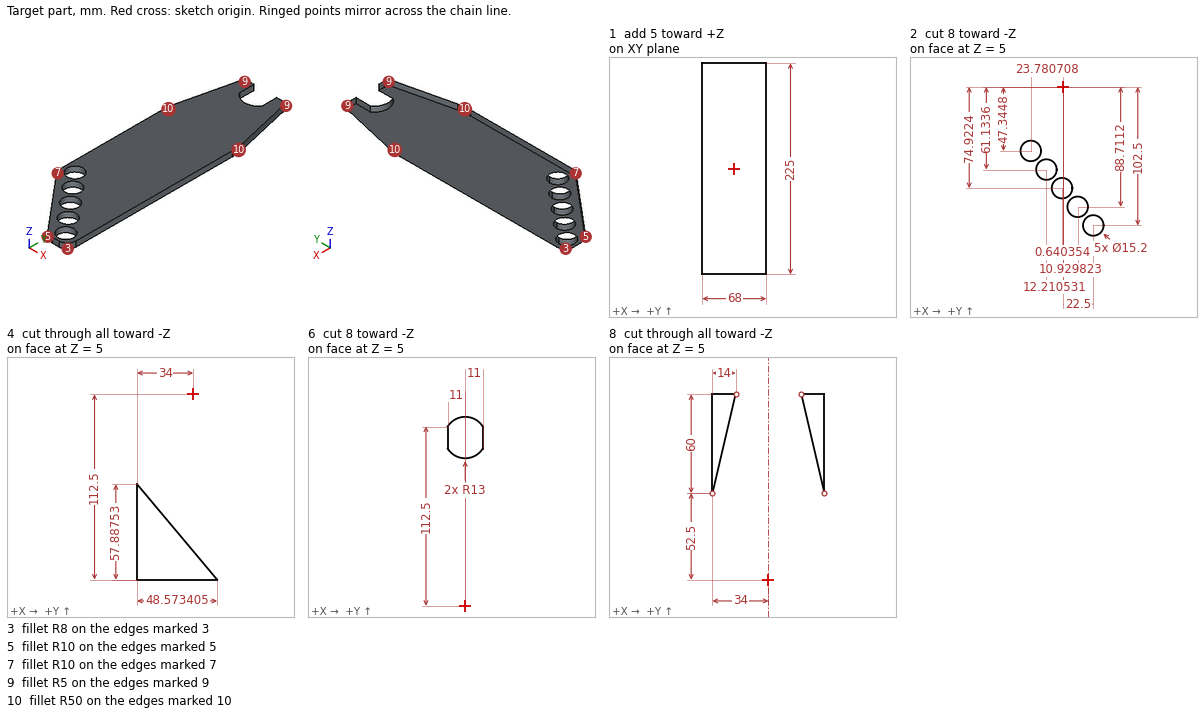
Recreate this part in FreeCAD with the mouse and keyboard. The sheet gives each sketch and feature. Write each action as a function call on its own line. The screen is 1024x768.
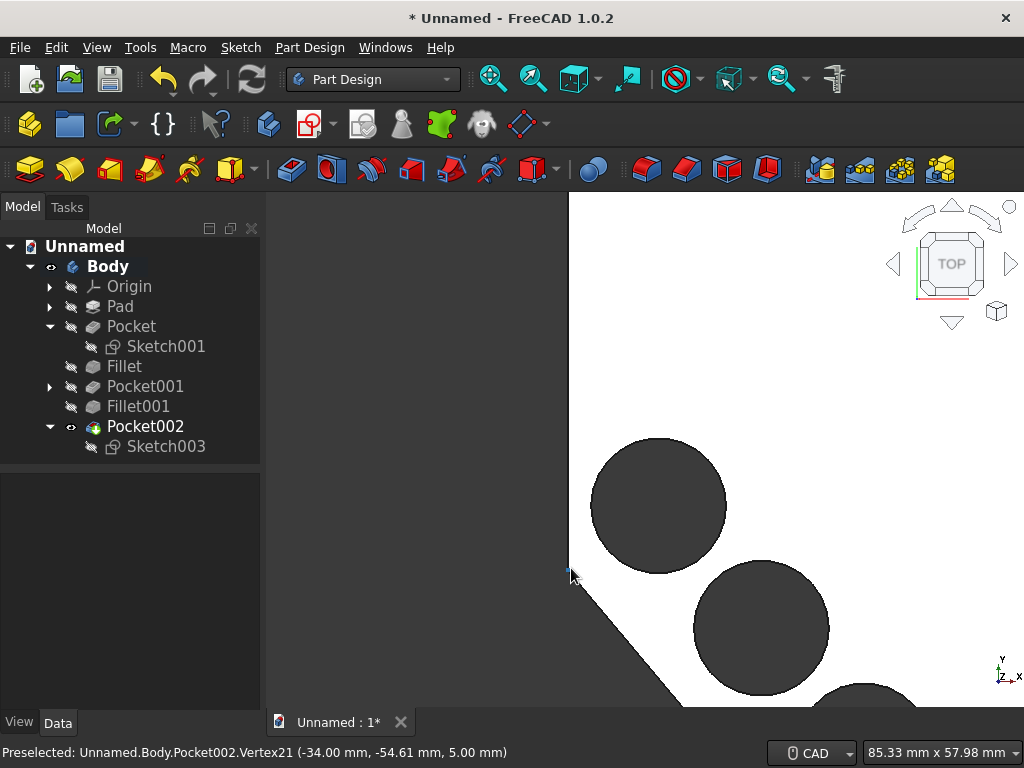
key(v)
key(f)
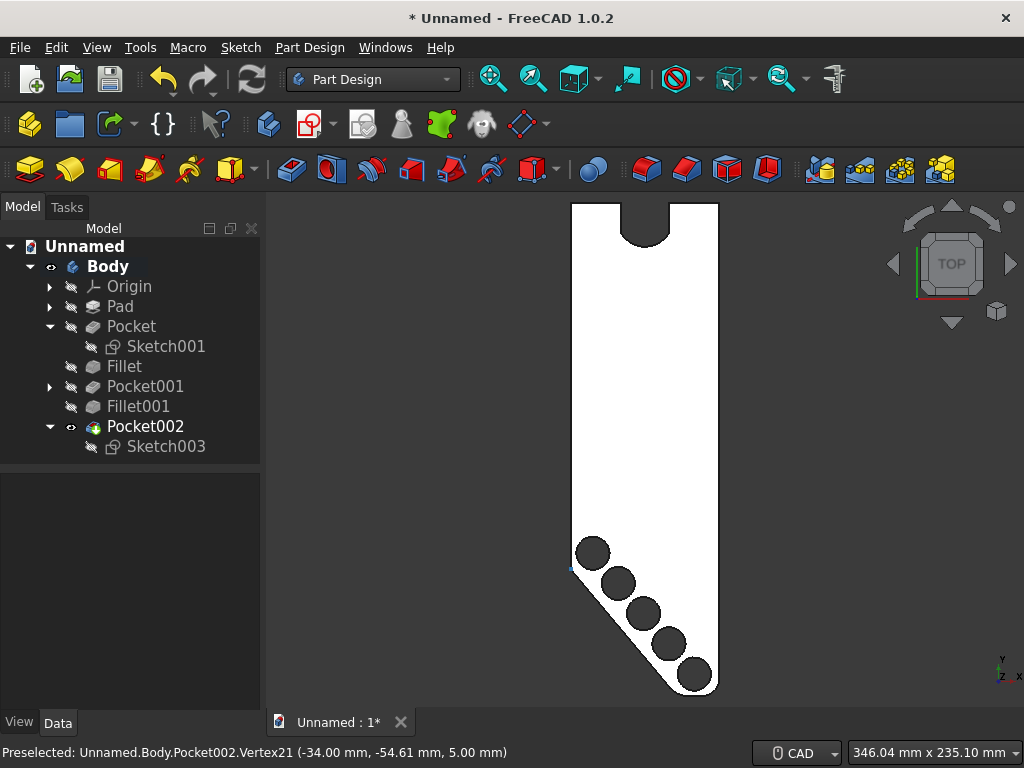
key(0)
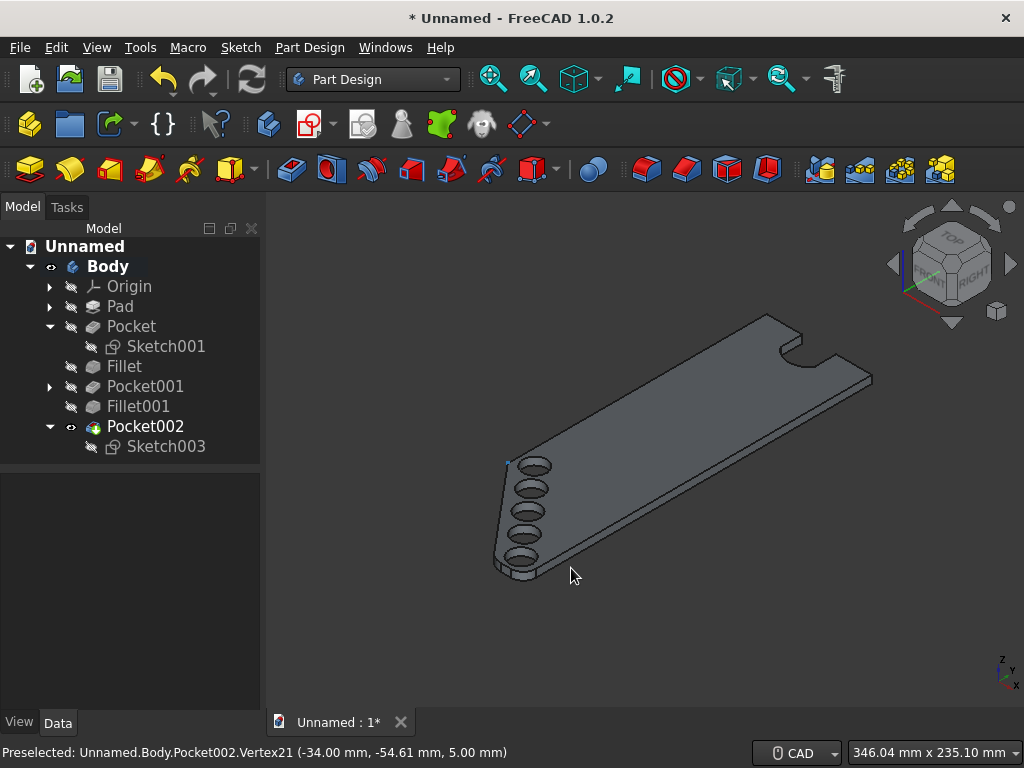
scroll(508, 467, up, 7)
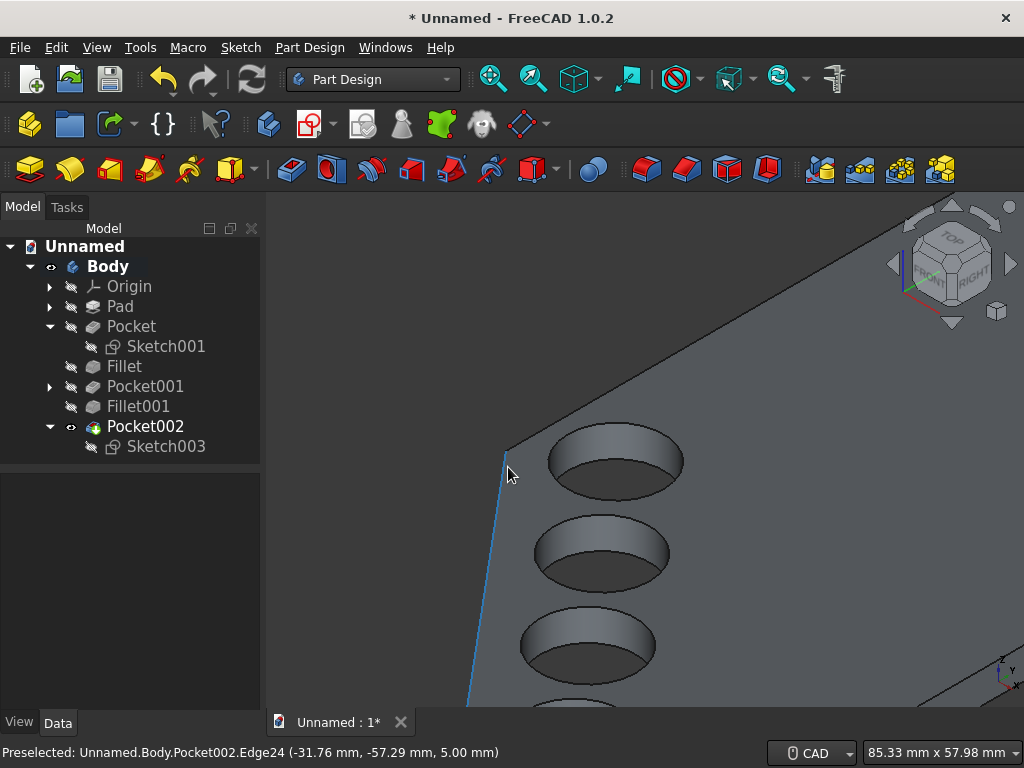
key(v)
key(f)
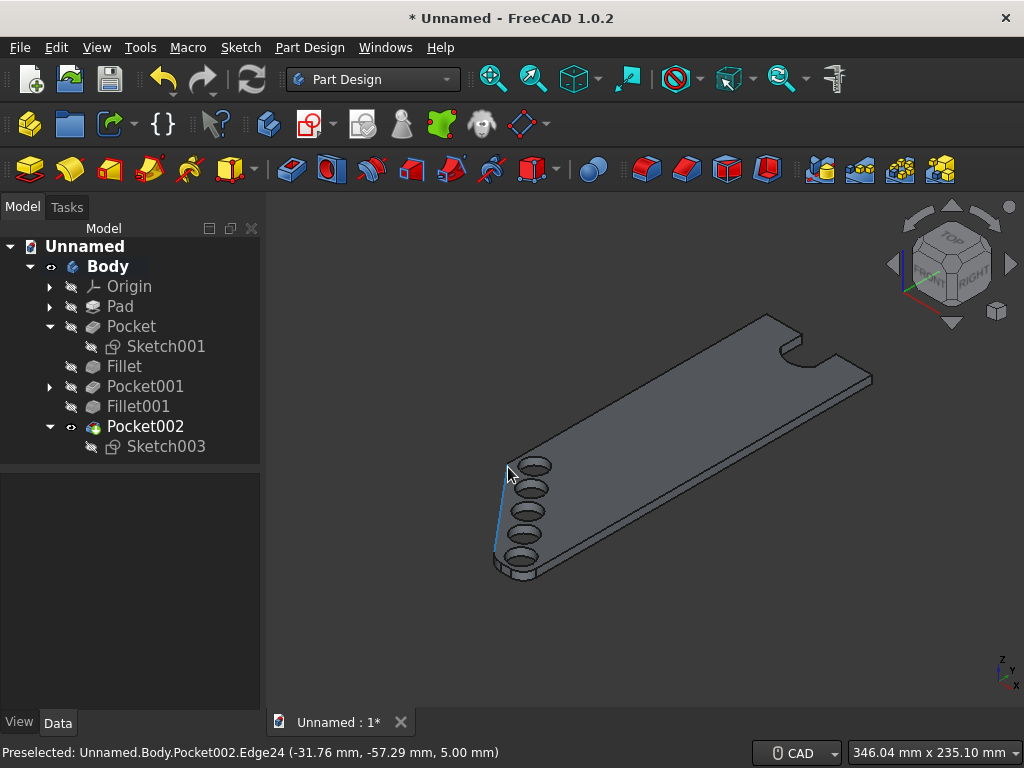
key(1)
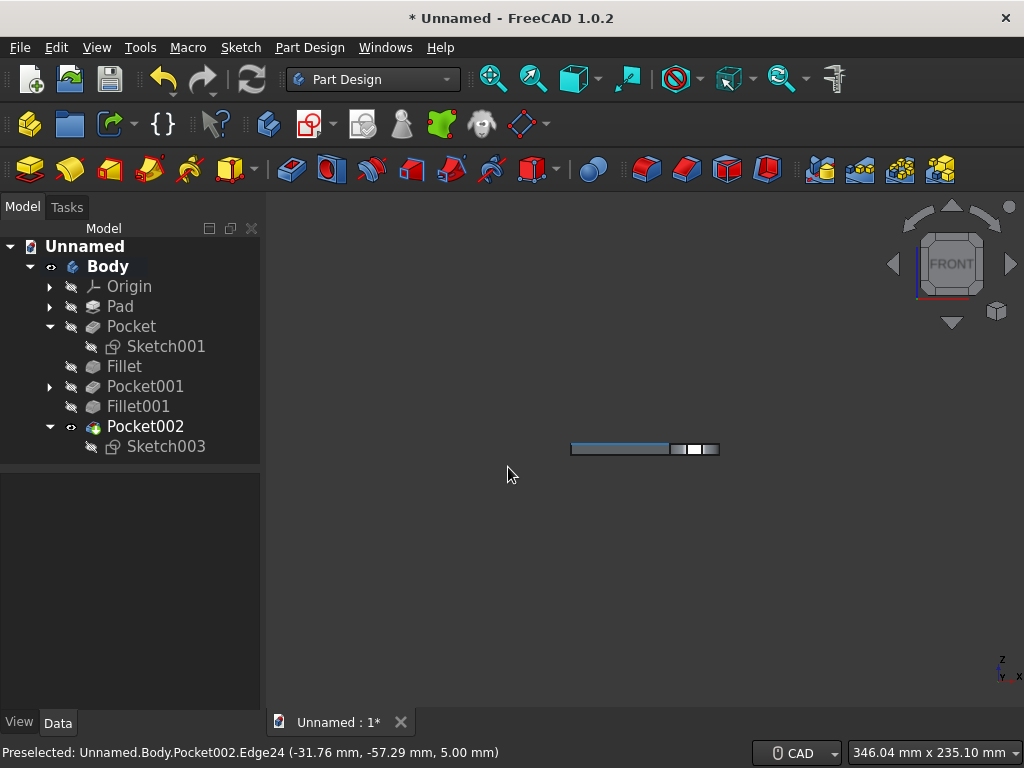
key(v)
key(f)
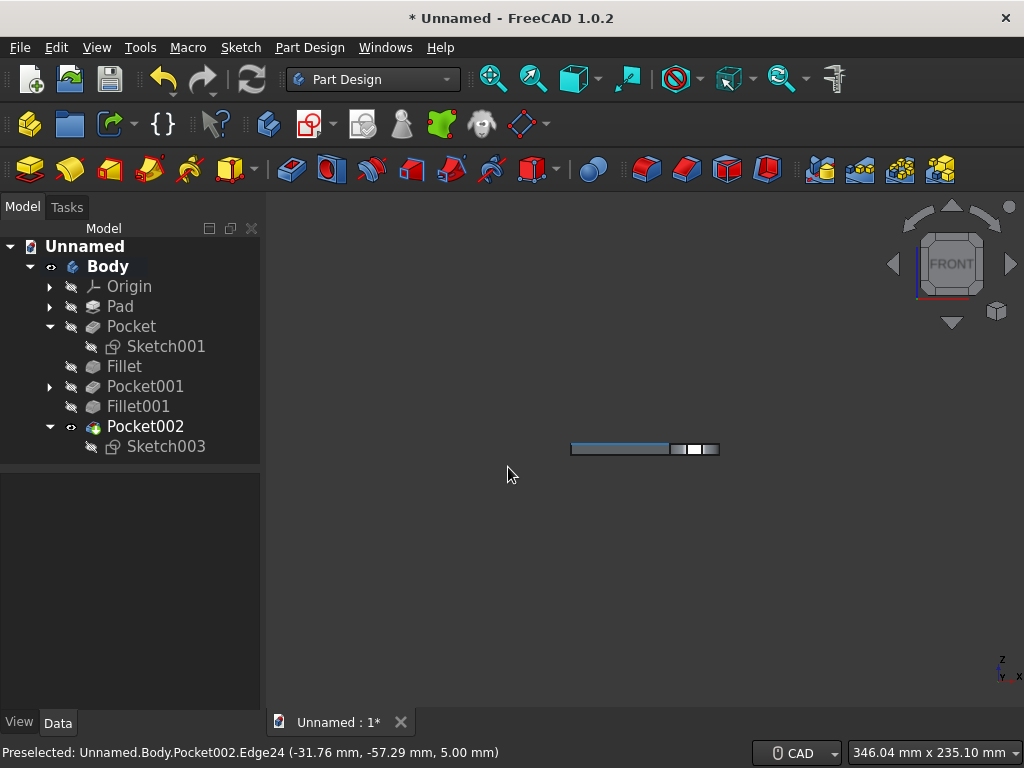
scroll(571, 449, up, 7)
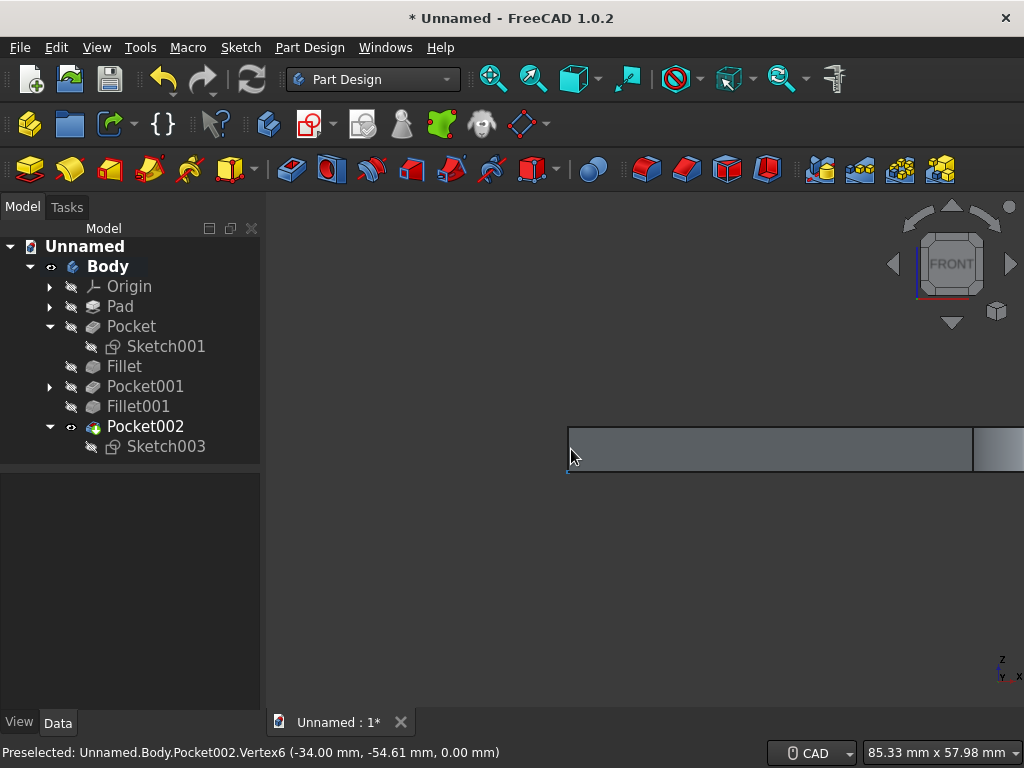
key(v)
key(f)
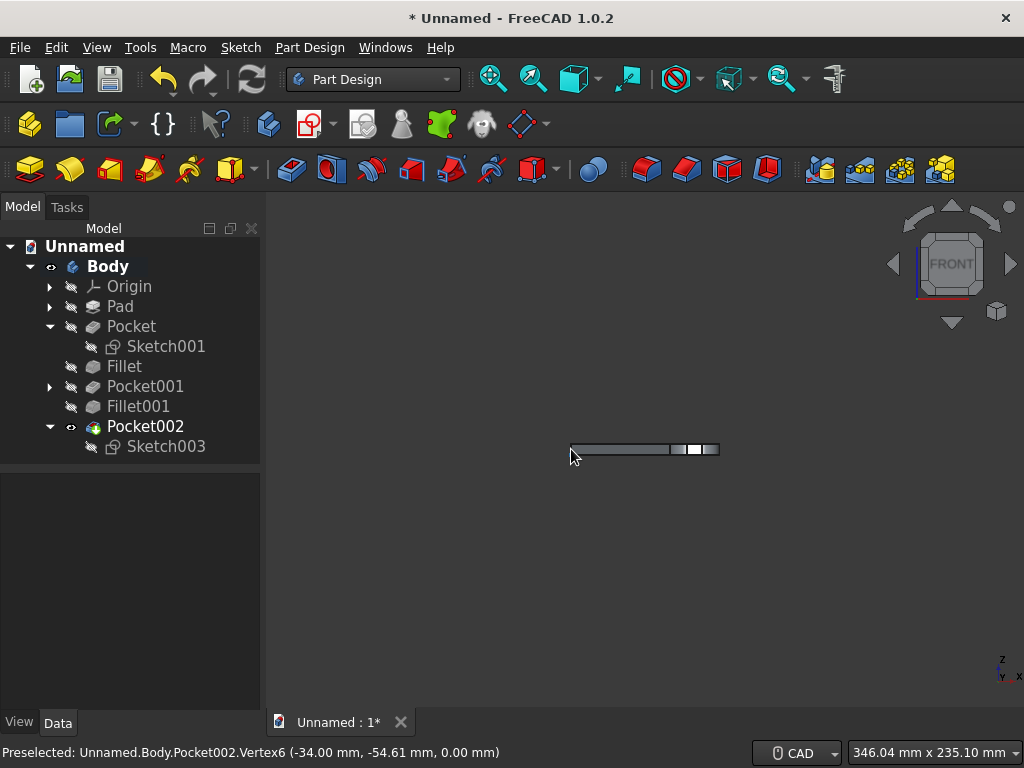
key(3)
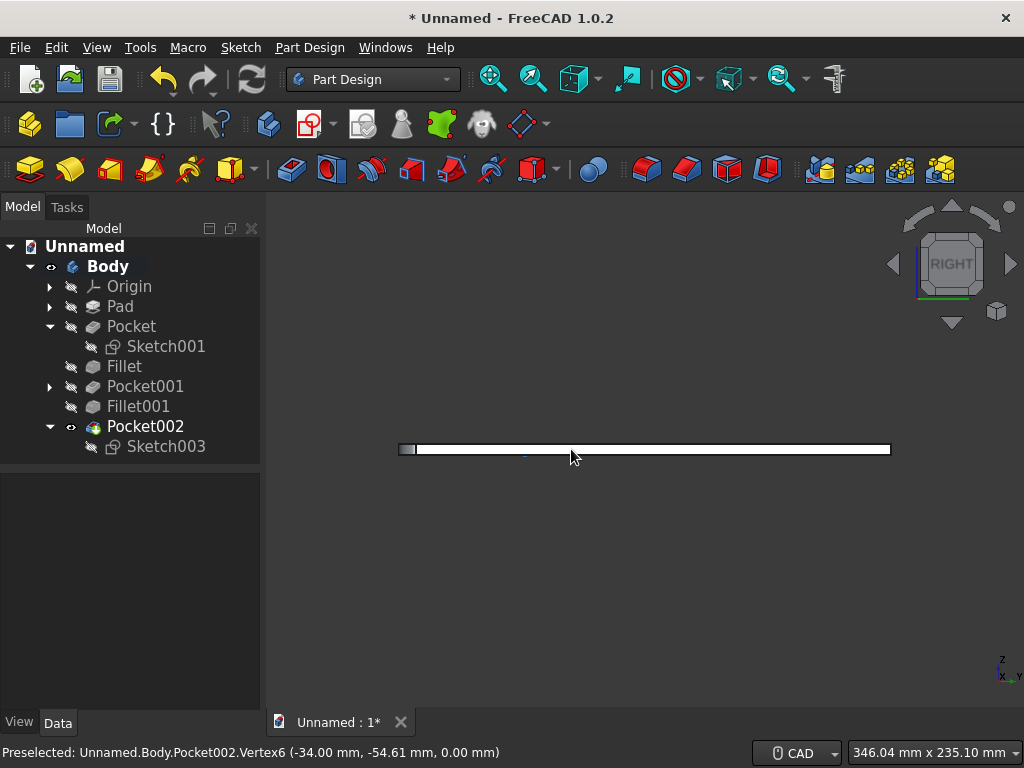
scroll(525, 448, up, 7)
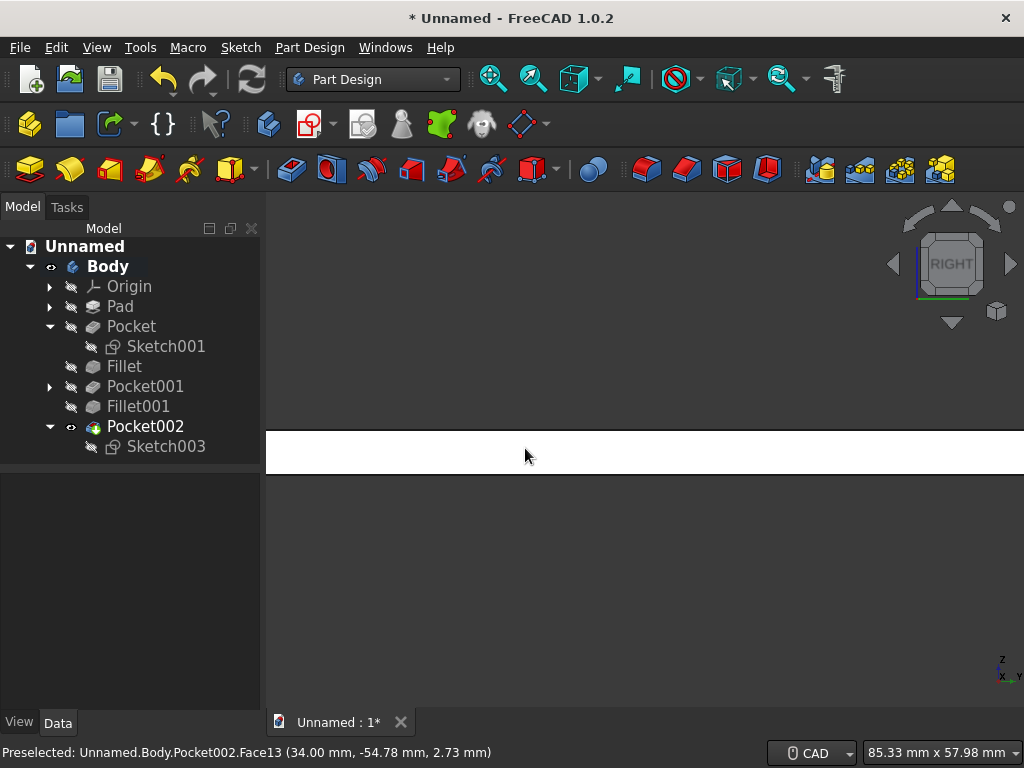
key(v)
key(f)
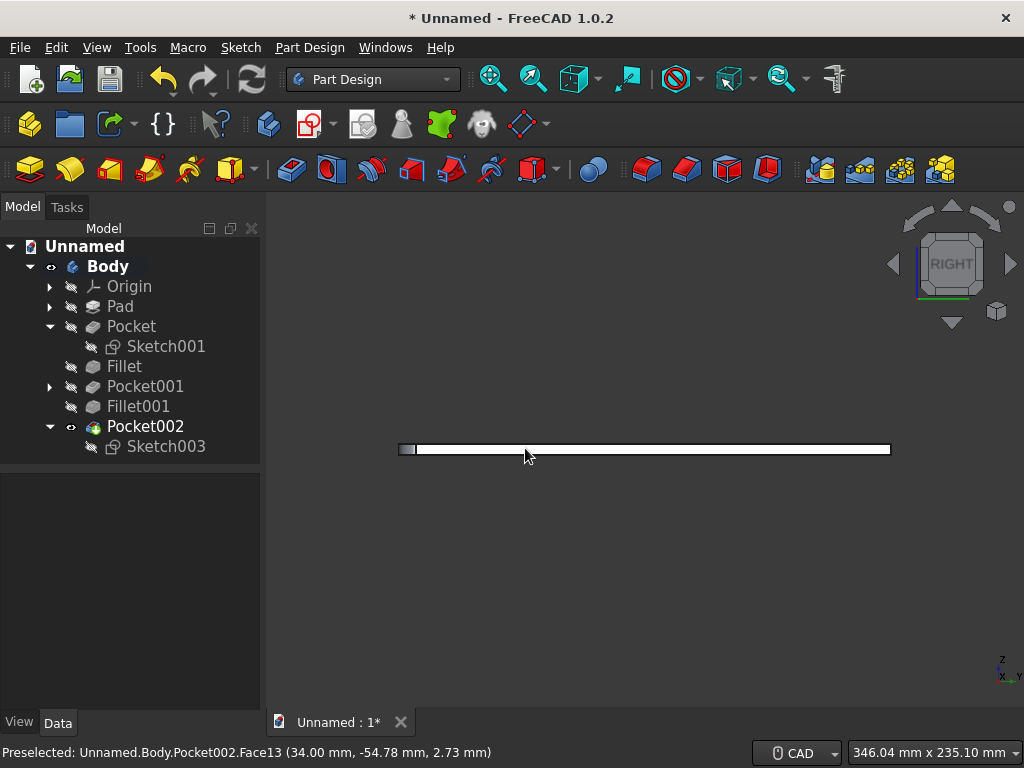
key(5)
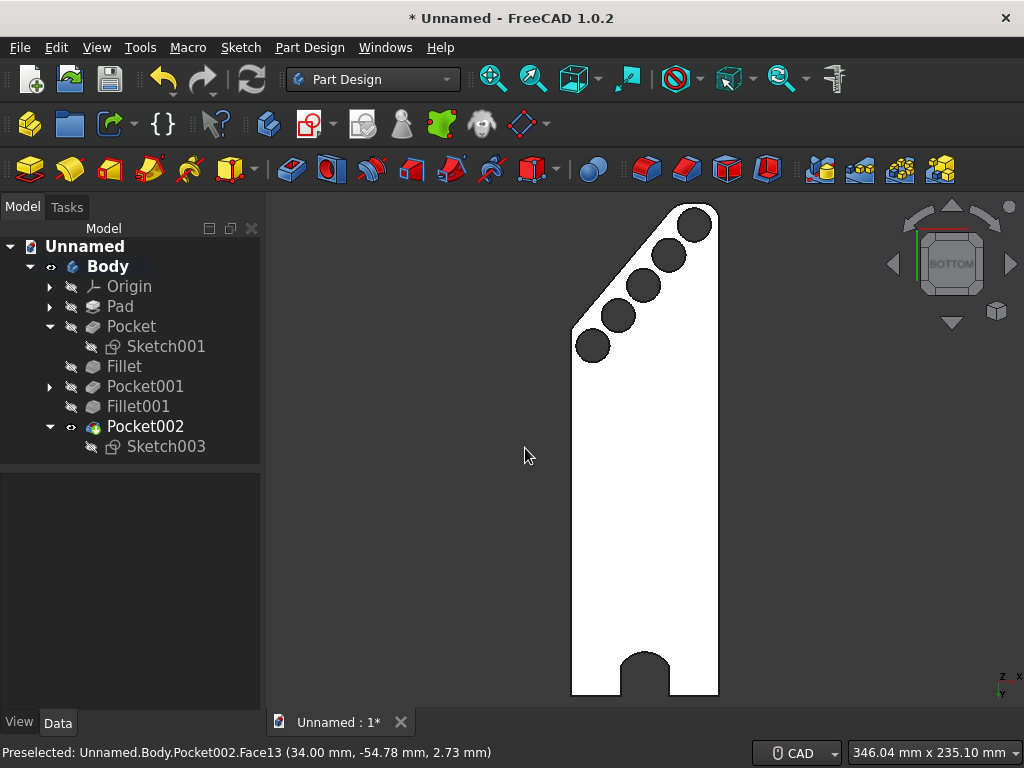
scroll(571, 329, up, 7)